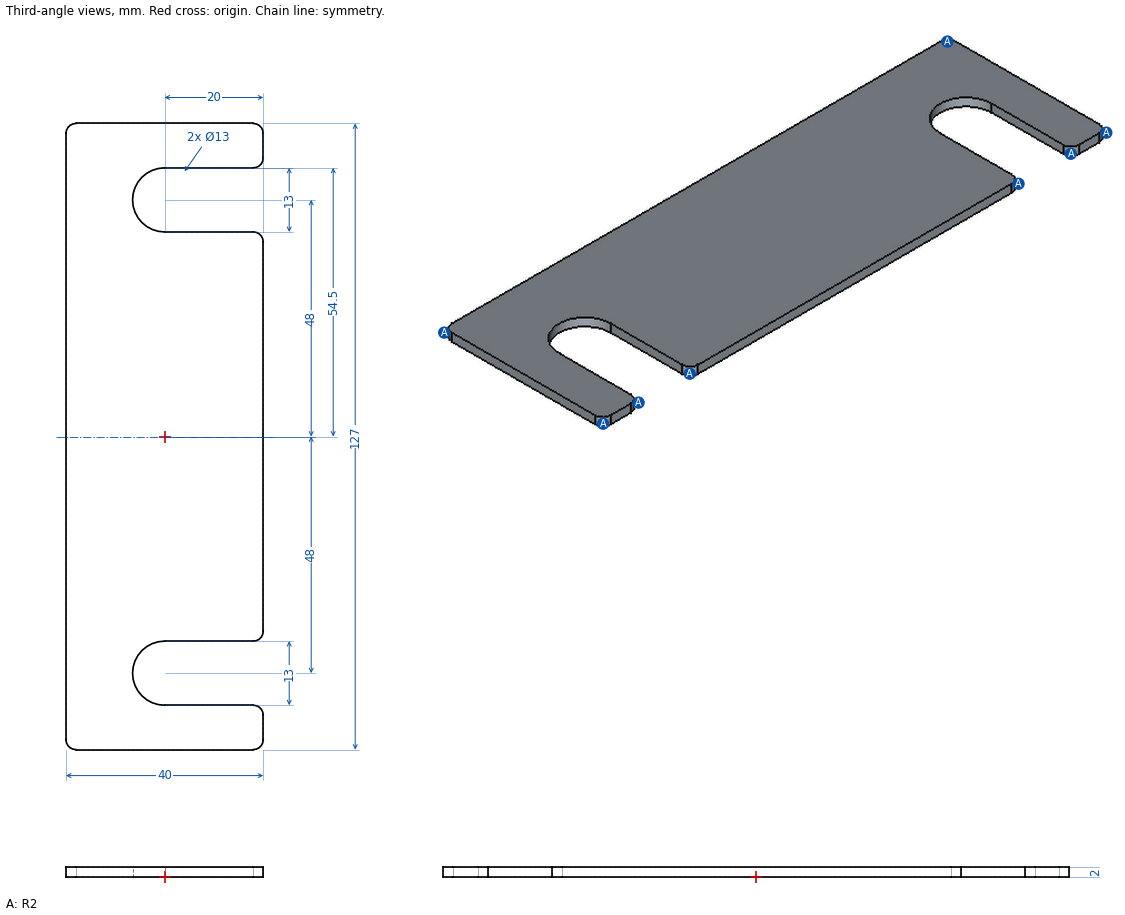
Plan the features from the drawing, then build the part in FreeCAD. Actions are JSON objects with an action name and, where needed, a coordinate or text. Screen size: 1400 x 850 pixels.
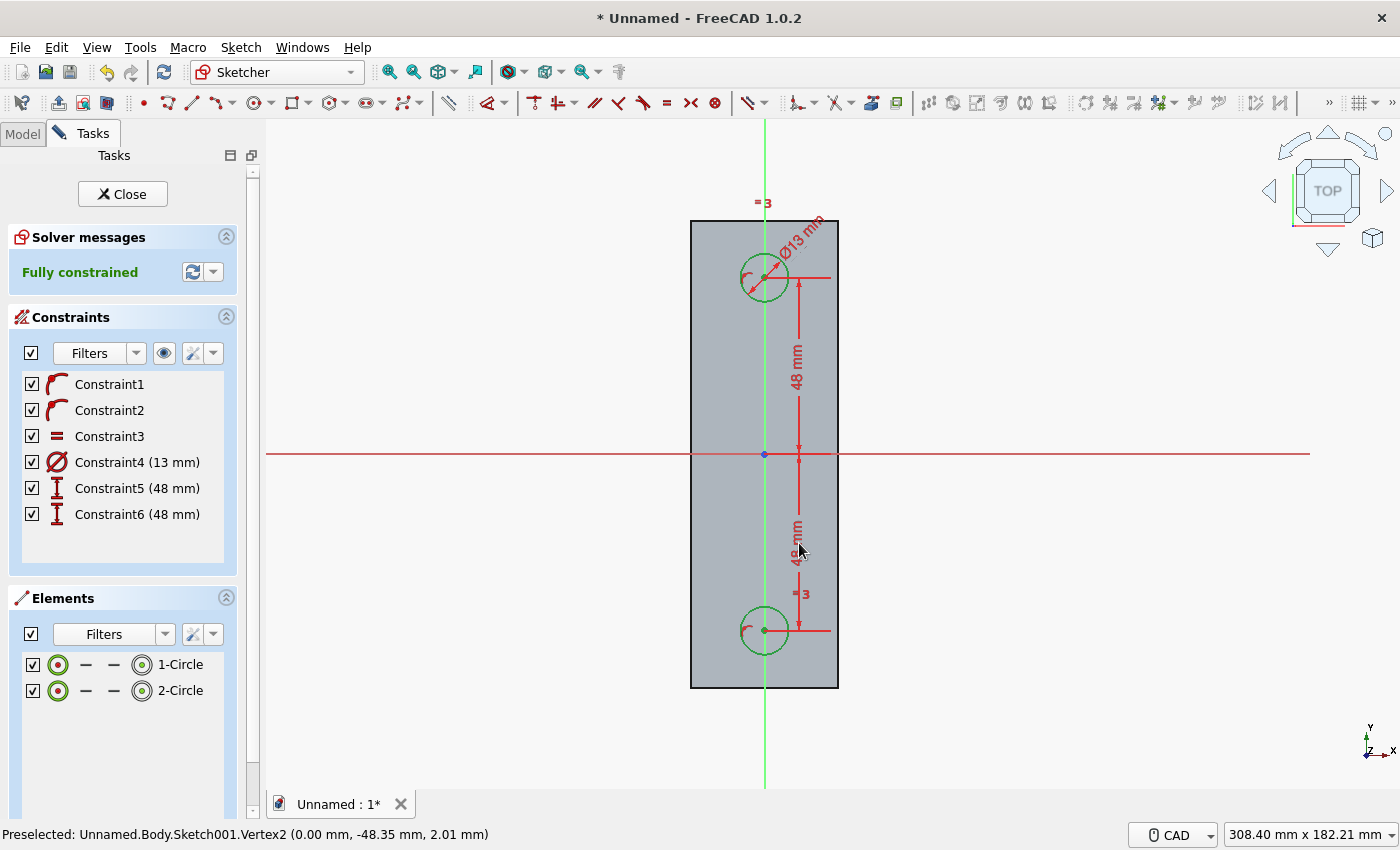
{"action": "left_click", "coordinate": [123, 194]}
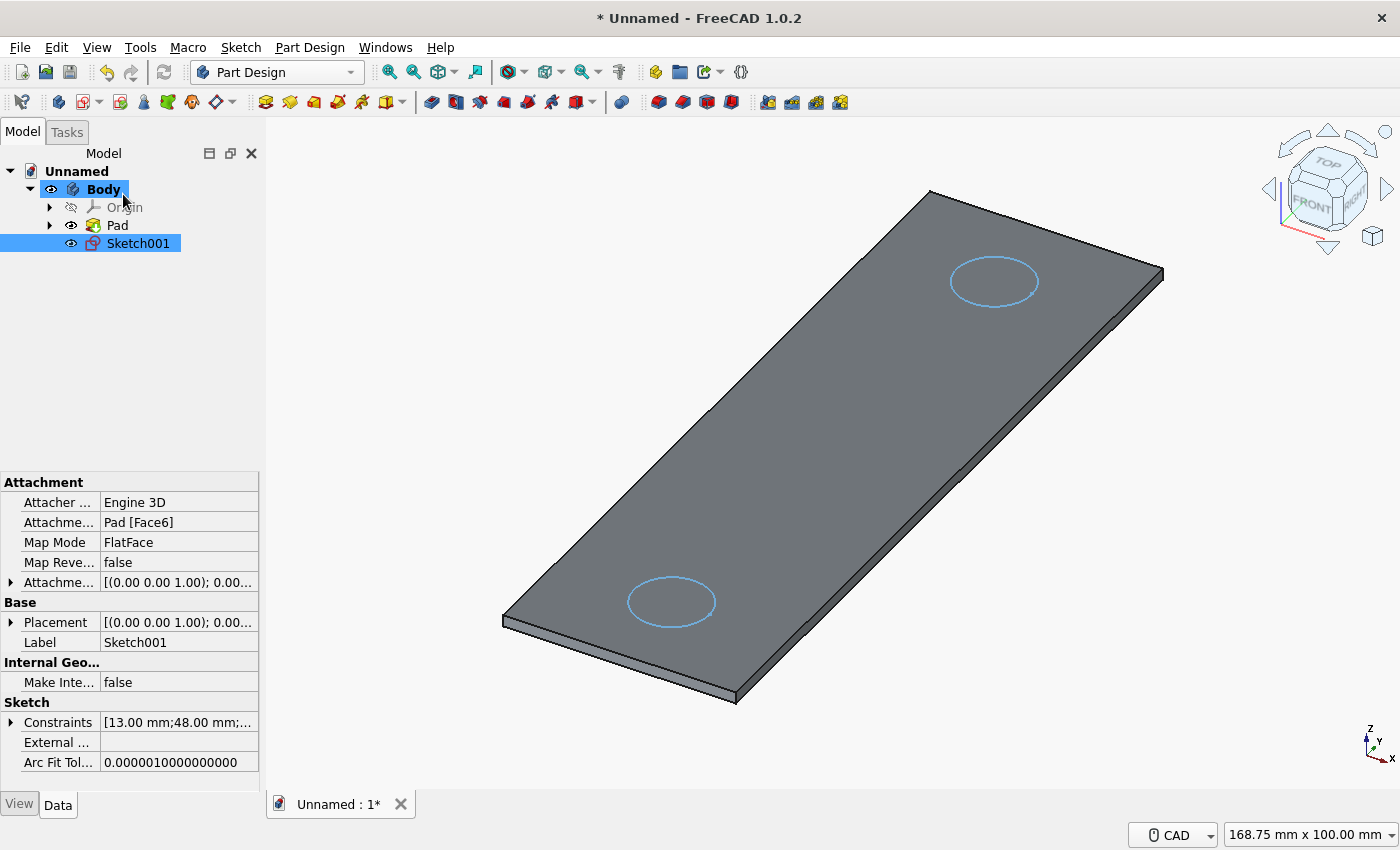
{"action": "left_click", "coordinate": [432, 102]}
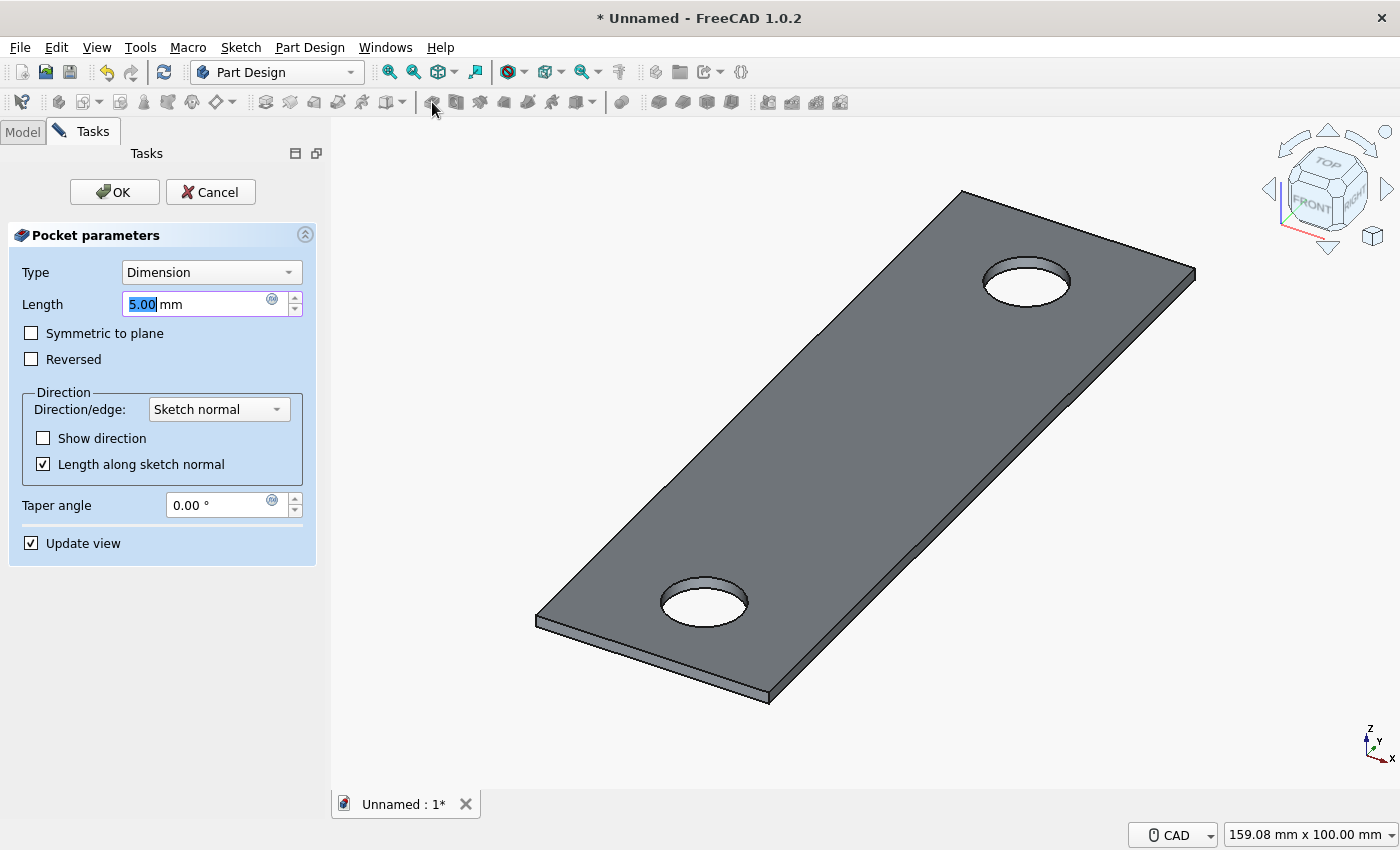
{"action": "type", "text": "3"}
{"action": "key", "text": "Tab"}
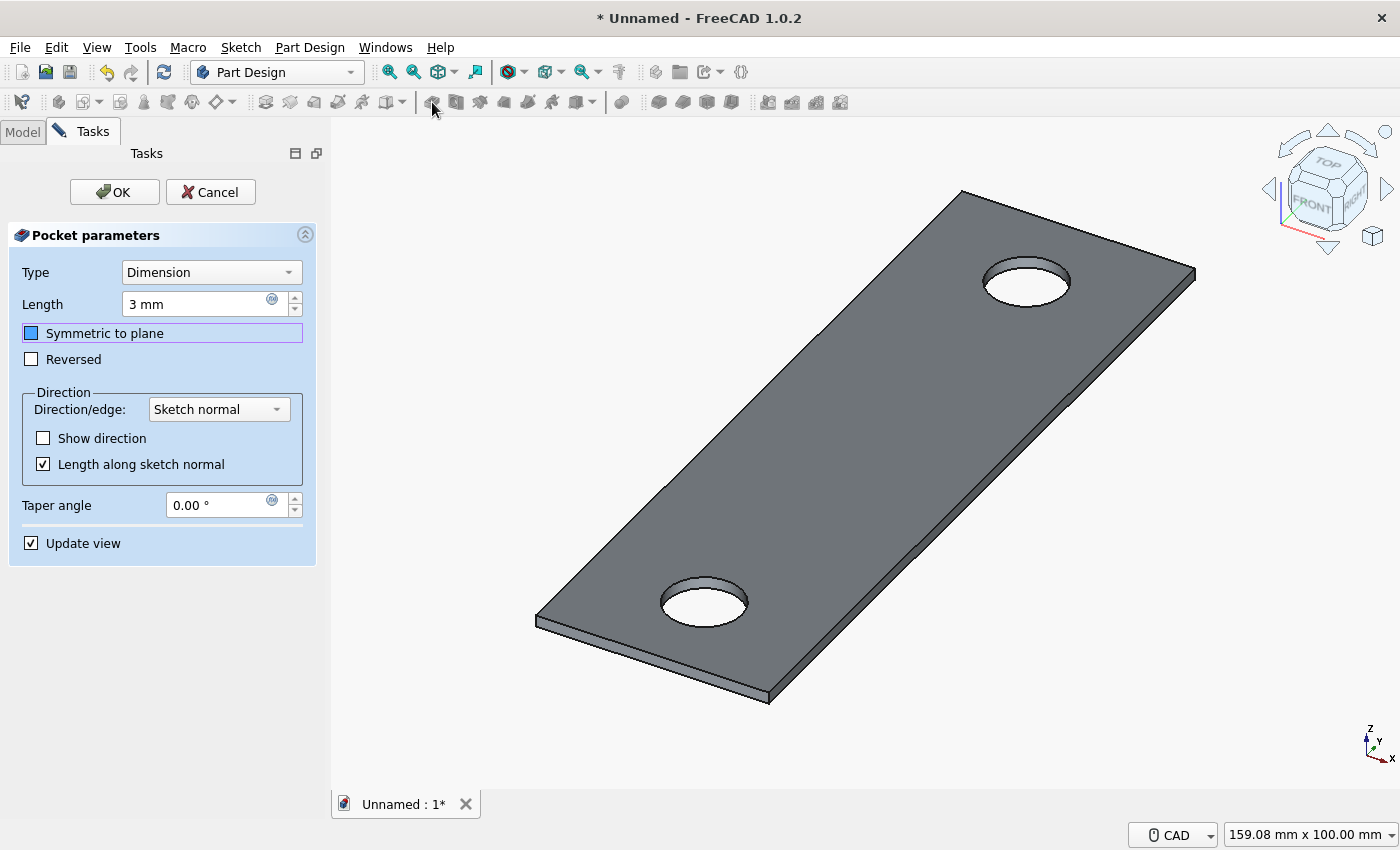
{"action": "left_click", "coordinate": [115, 192]}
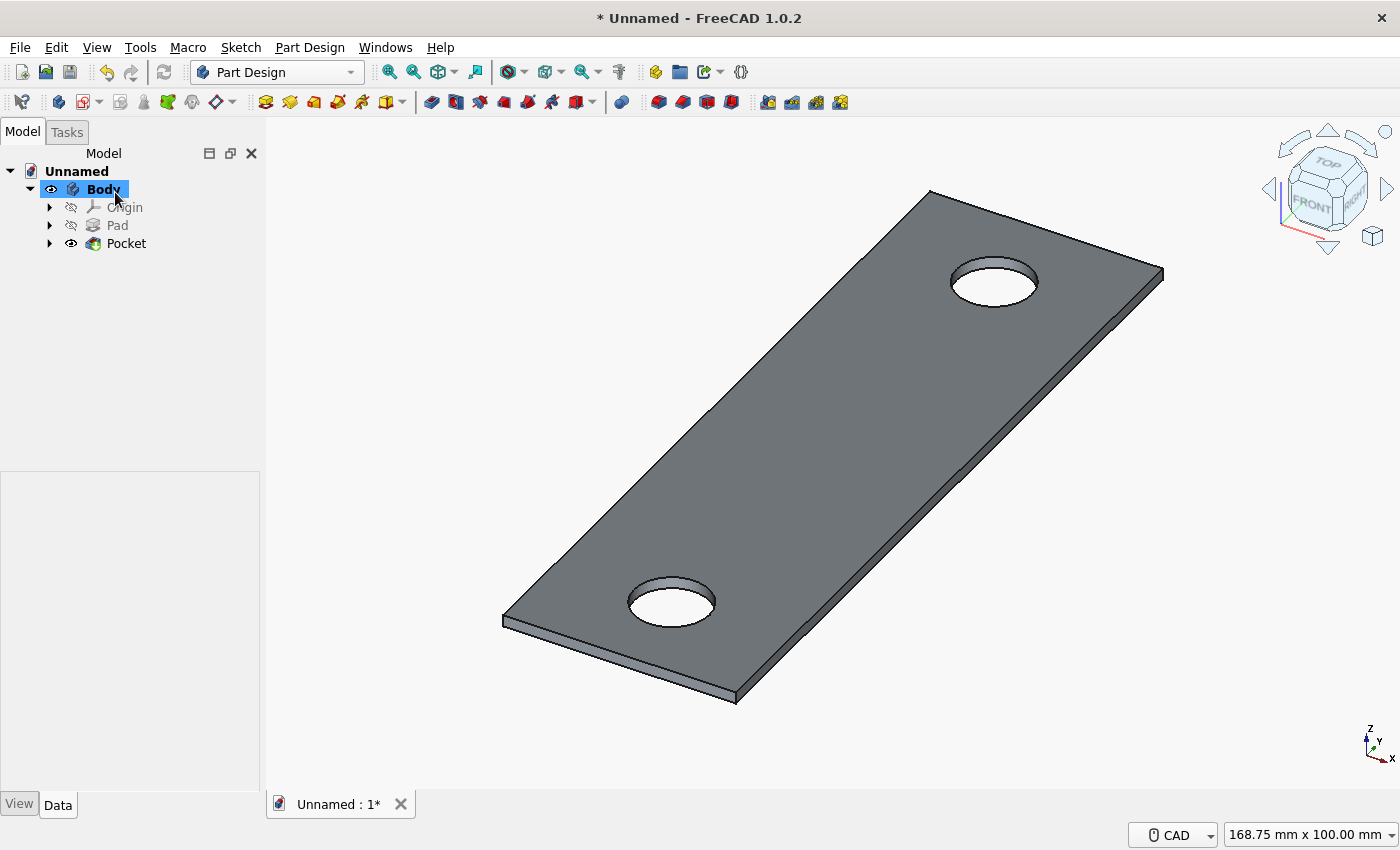
{"action": "left_click", "coordinate": [894, 380]}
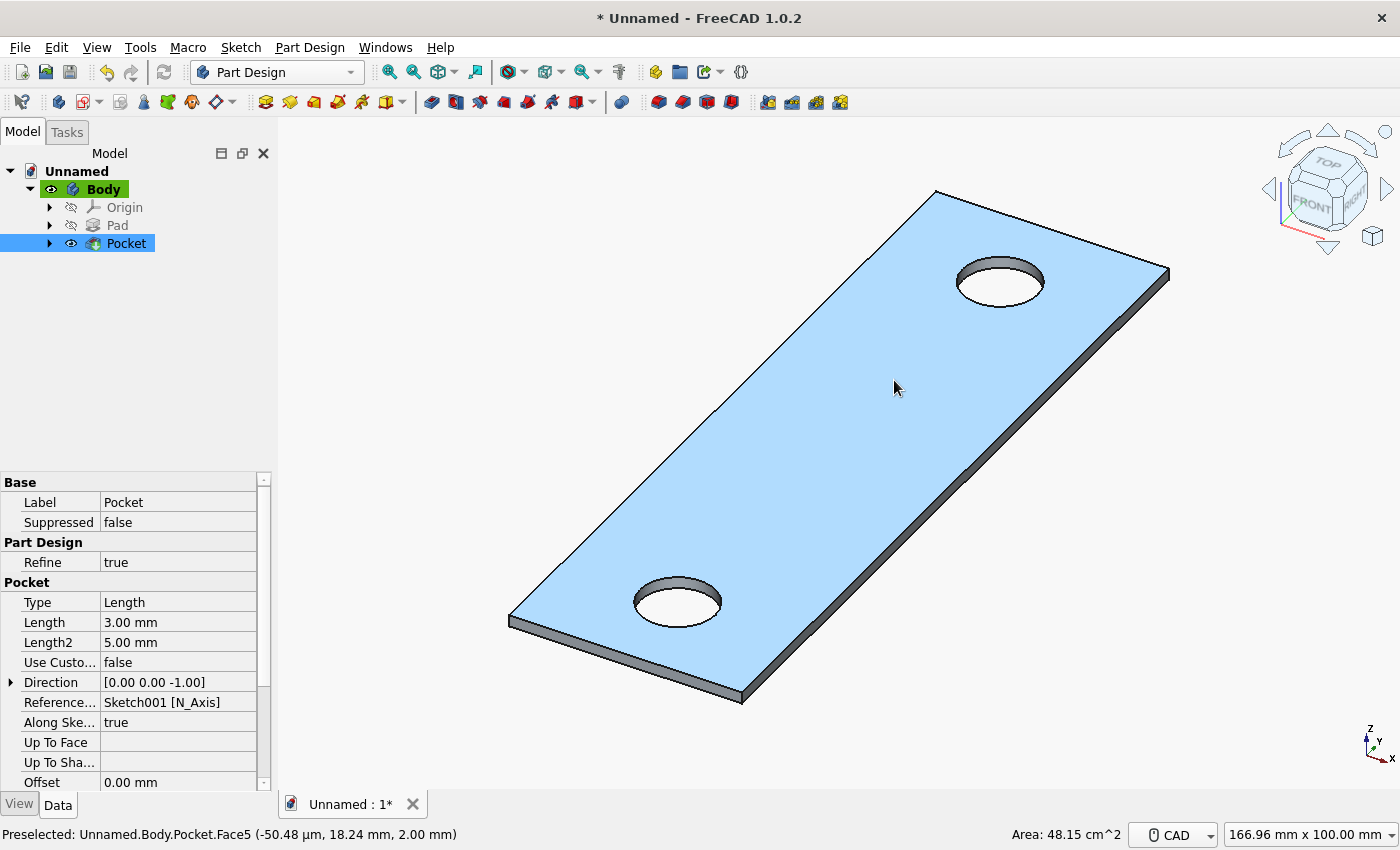
{"action": "left_click", "coordinate": [84, 102]}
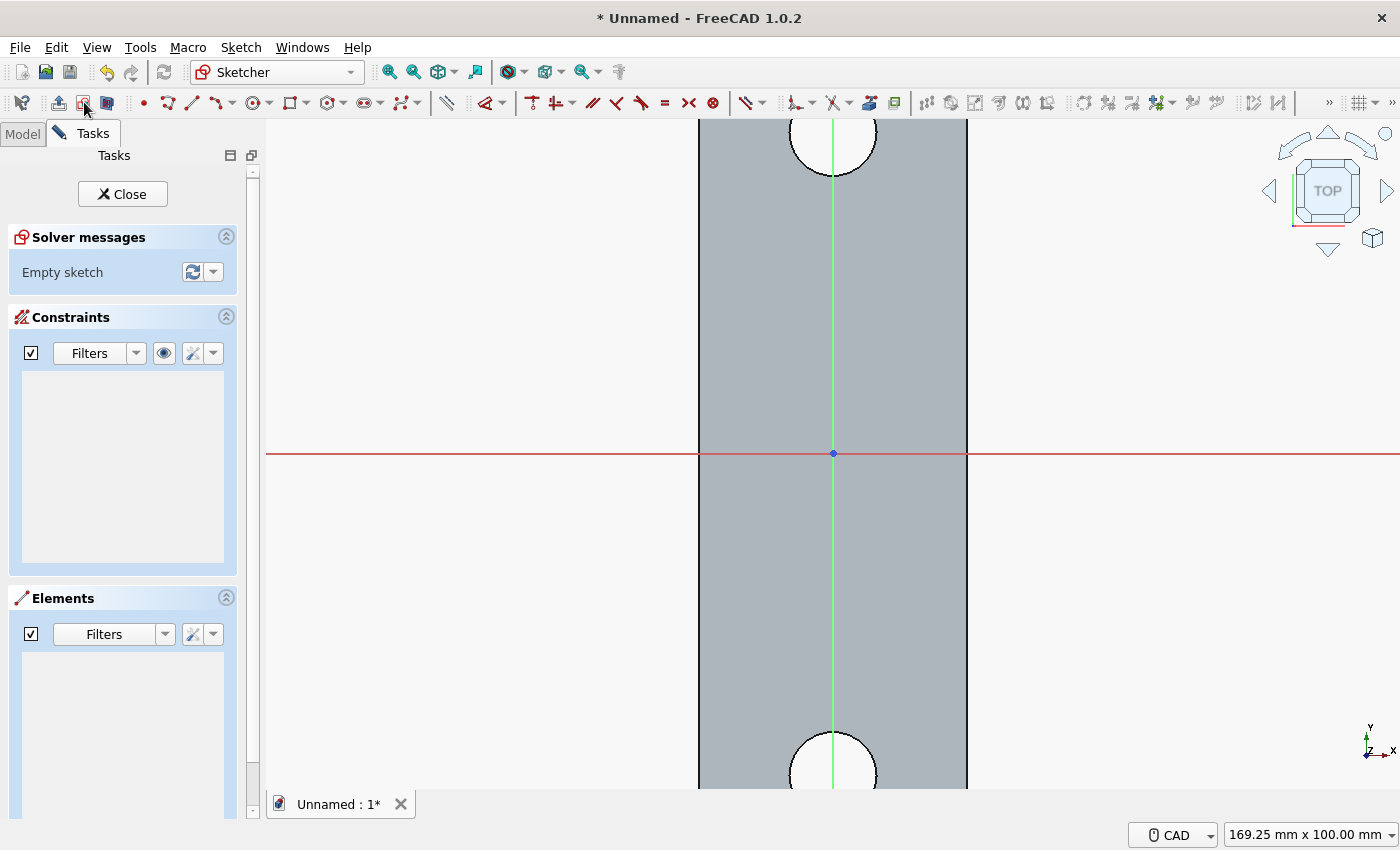
{"action": "scroll", "coordinate": [600, 454], "scroll_direction": "down", "scroll_amount": 3}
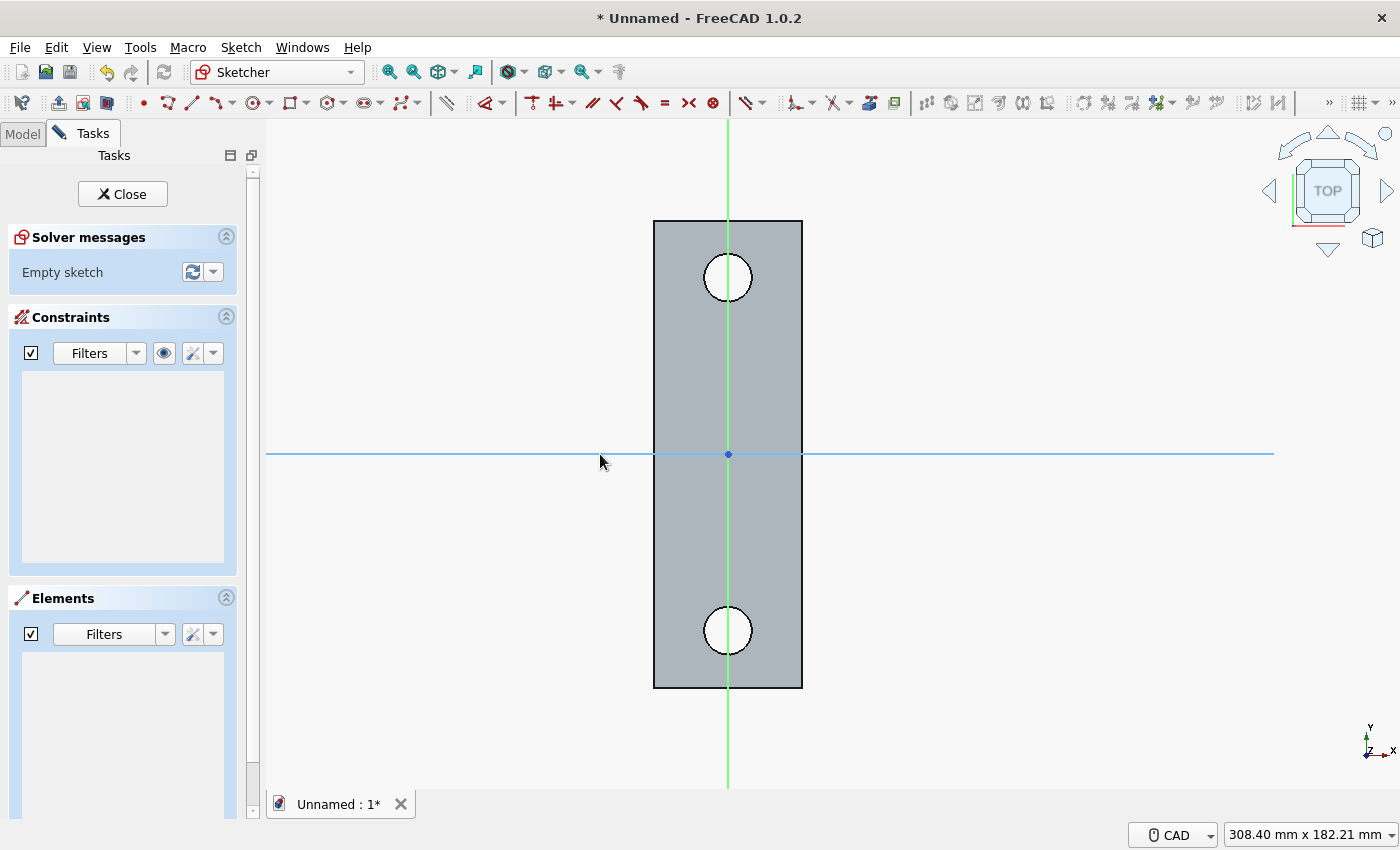
{"action": "left_click", "coordinate": [290, 104]}